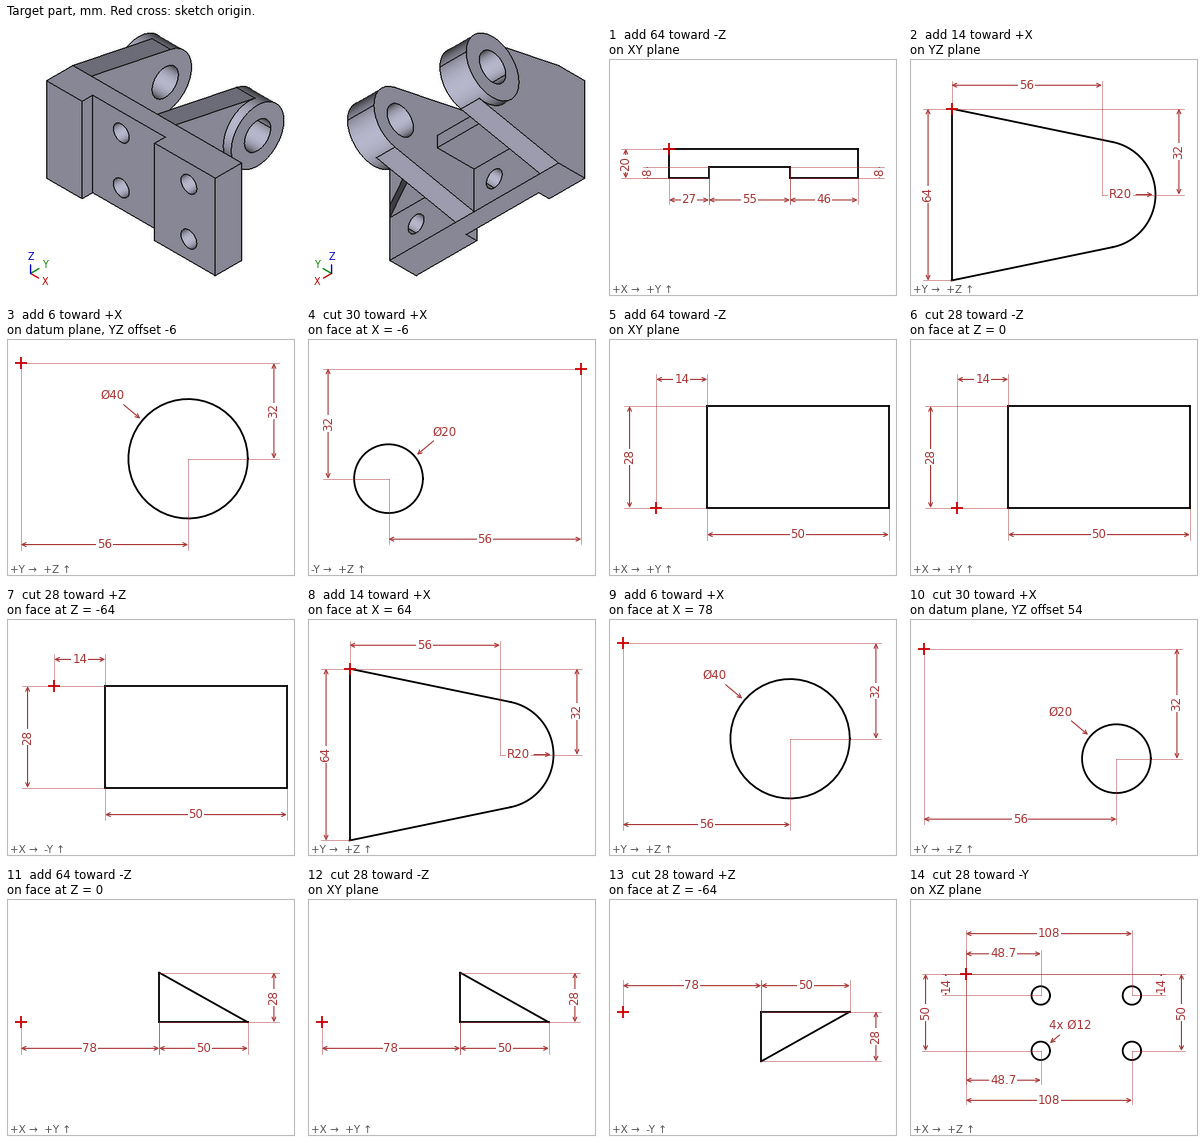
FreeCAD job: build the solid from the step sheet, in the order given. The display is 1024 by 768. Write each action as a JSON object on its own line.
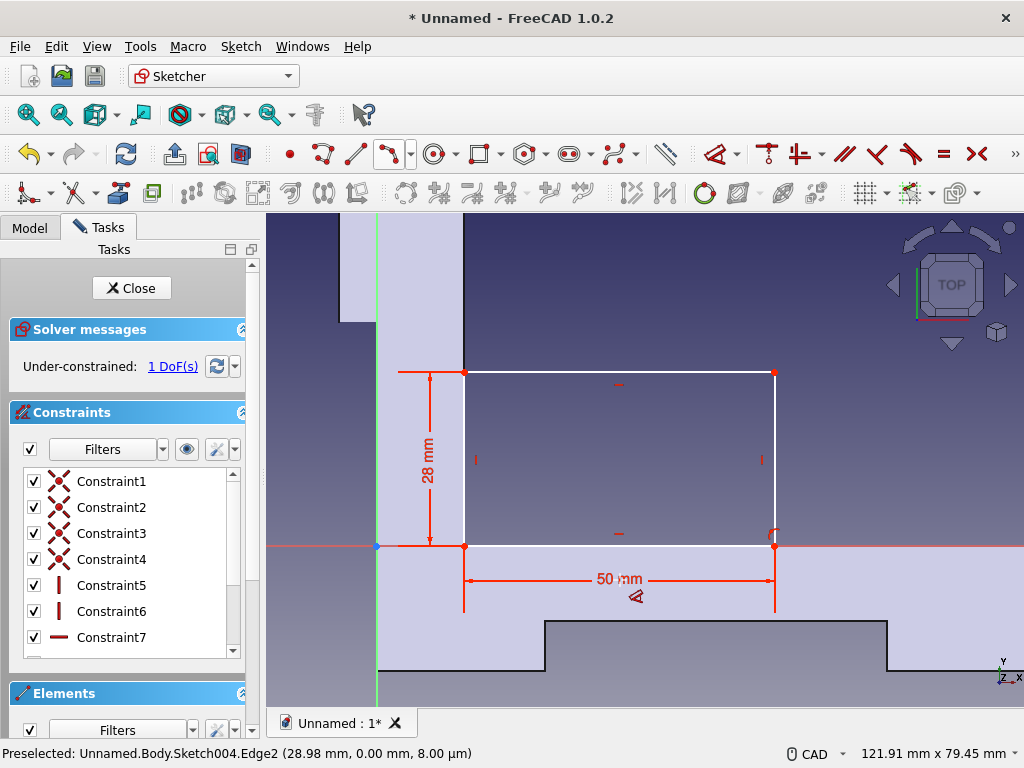
{"action": "left_click", "coordinate": [464, 372]}
{"action": "left_click", "coordinate": [420, 580]}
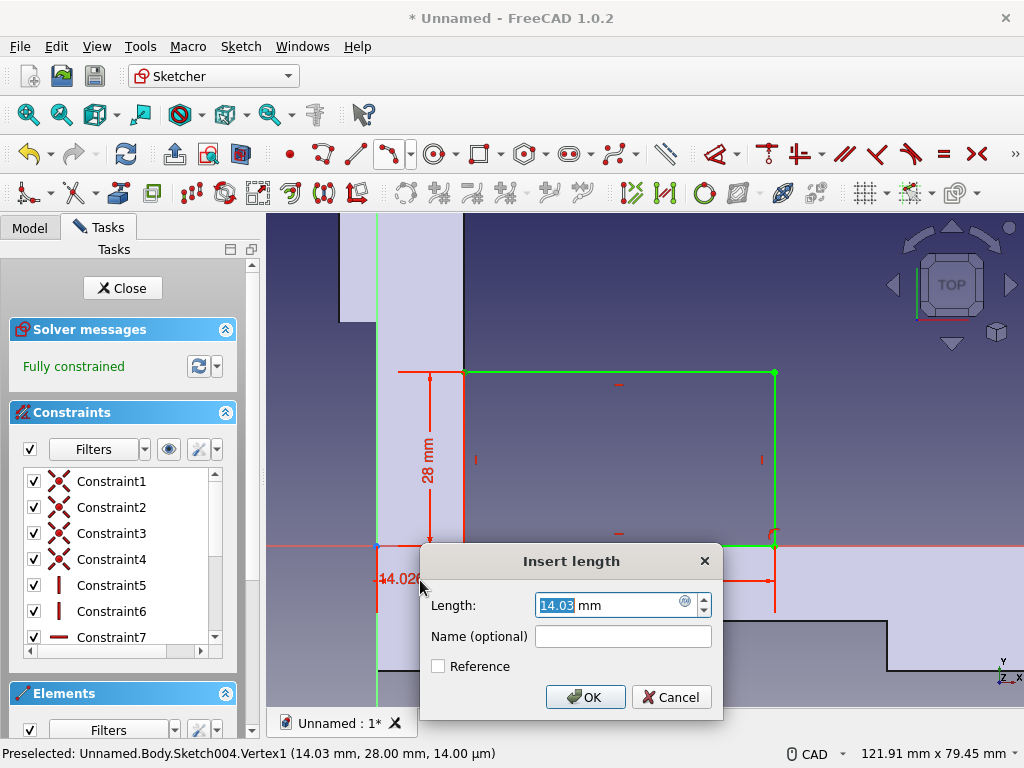
{"action": "type", "text": "14"}
{"action": "key", "text": "Return"}
{"action": "key", "text": "Escape"}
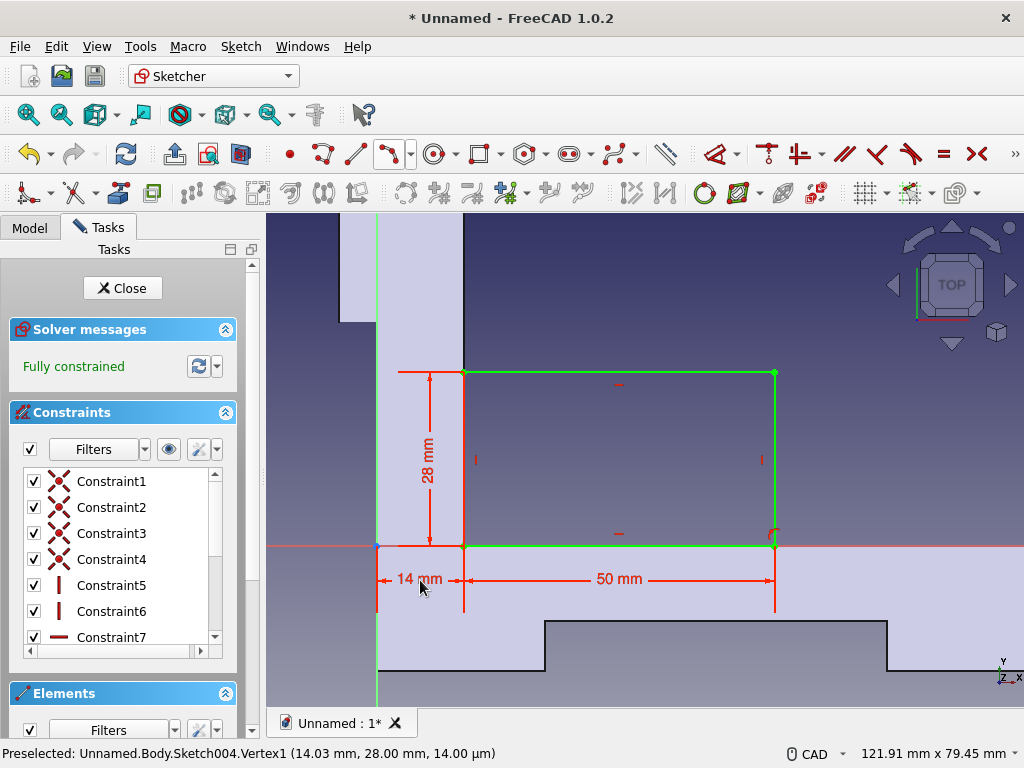
{"action": "left_click", "coordinate": [123, 288]}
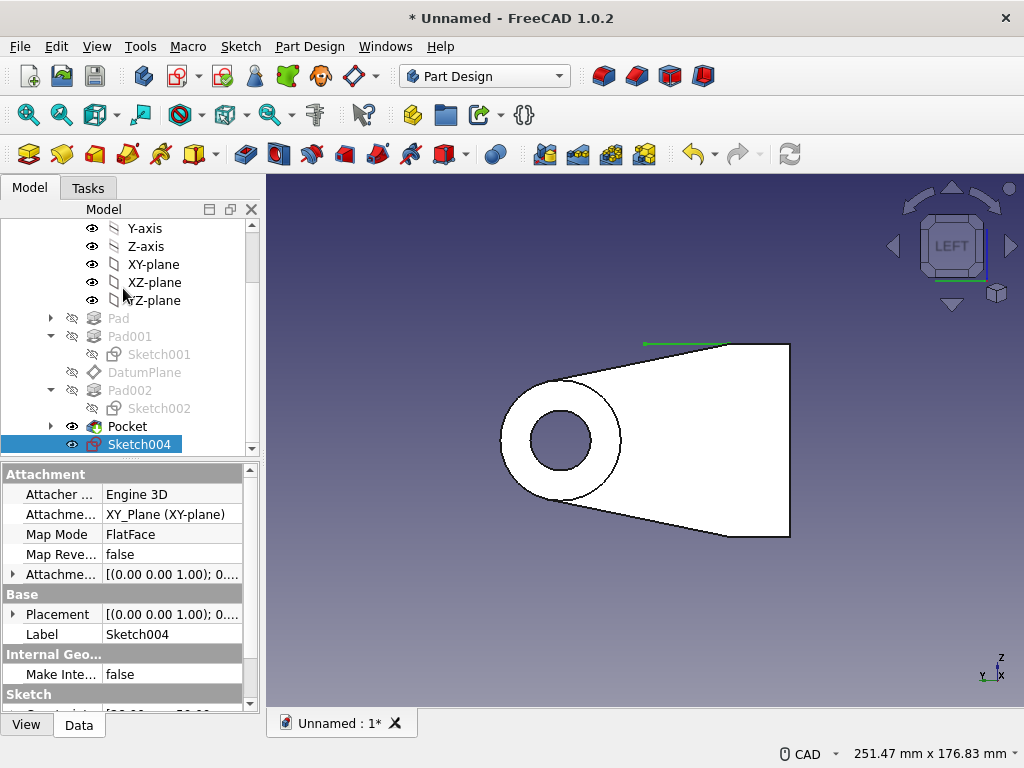
{"action": "left_click", "coordinate": [29, 154]}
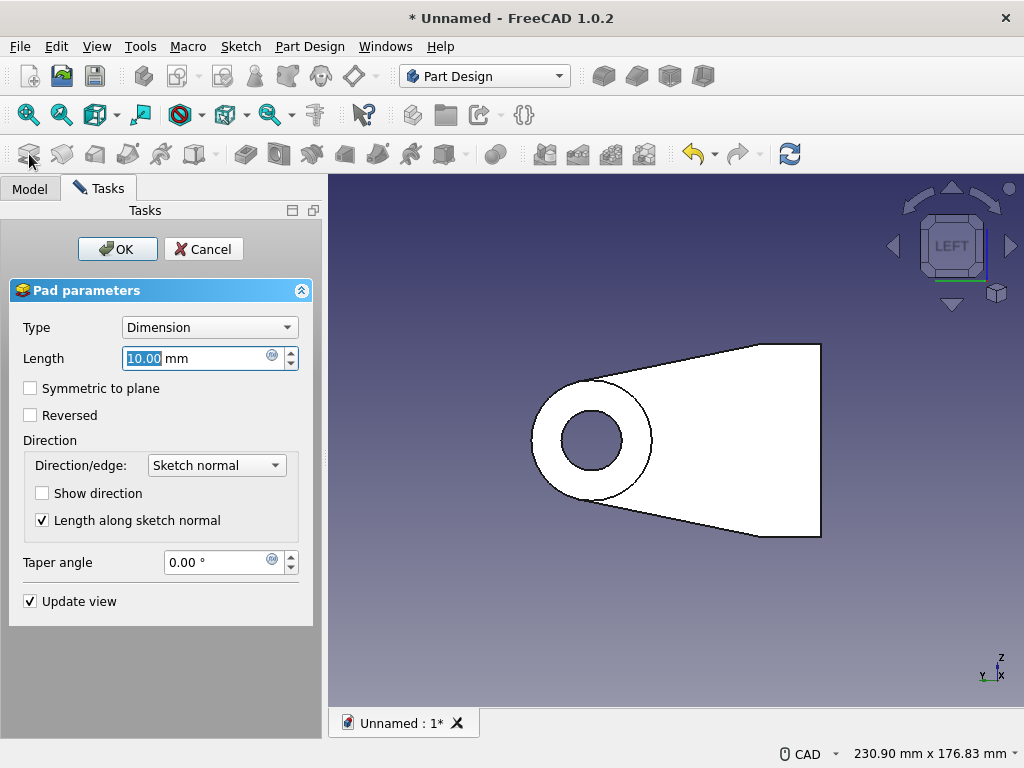
{"action": "type", "text": "64"}
{"action": "key", "text": "Tab"}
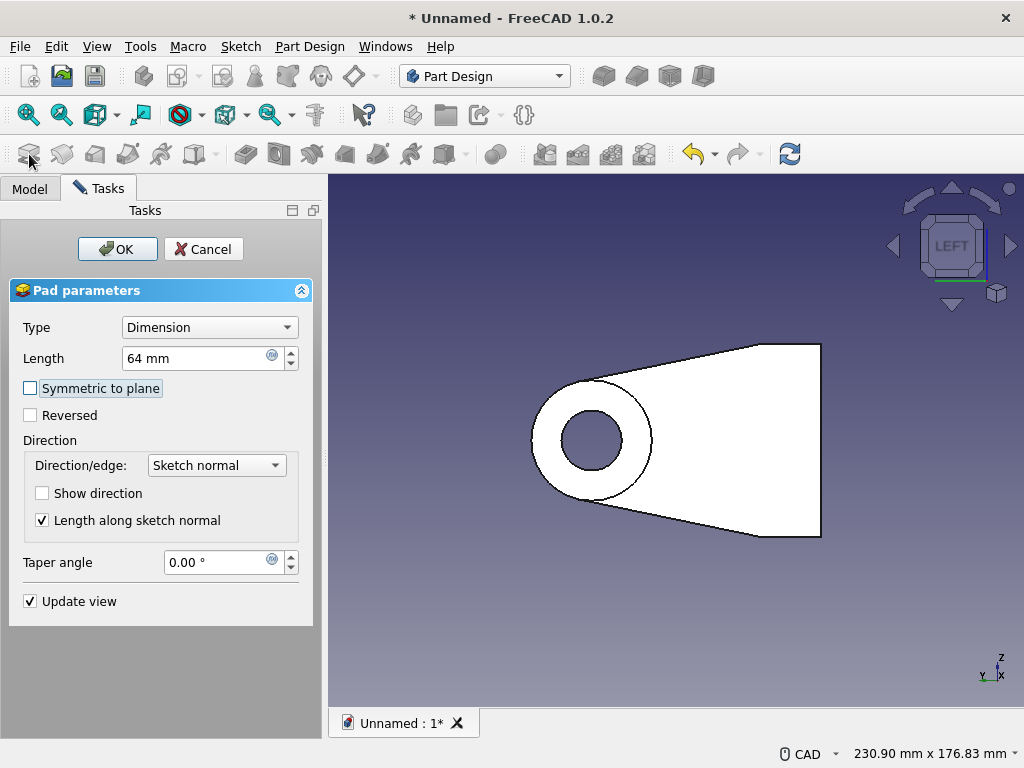
{"action": "left_click", "coordinate": [31, 415]}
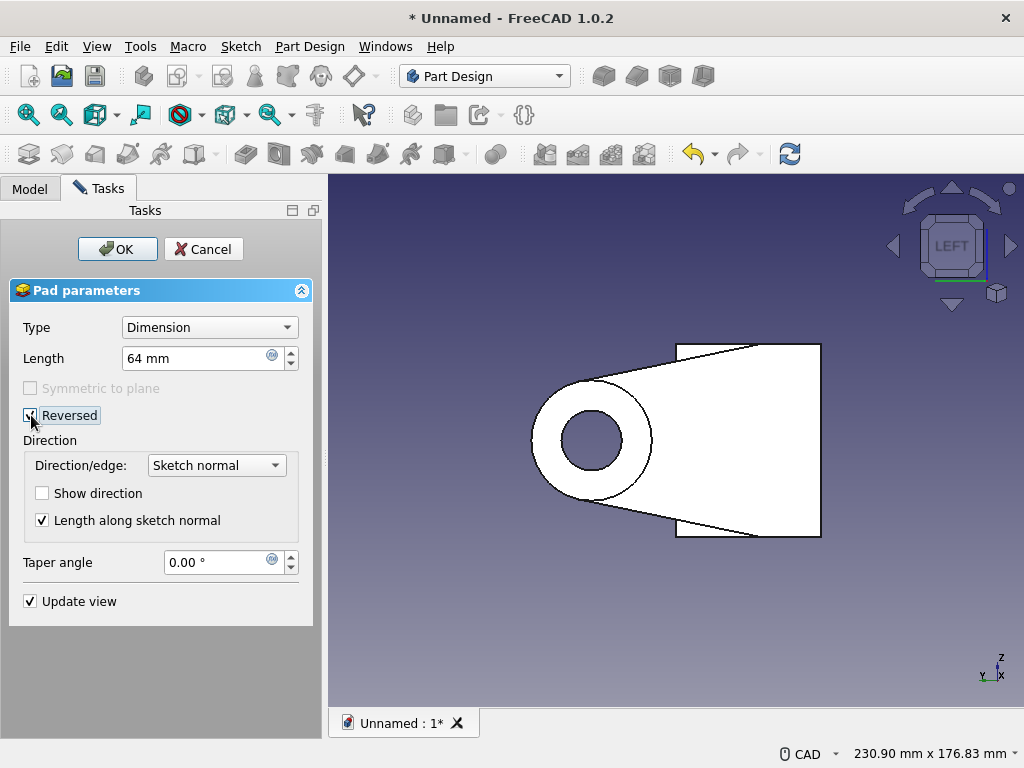
{"action": "left_click", "coordinate": [118, 249]}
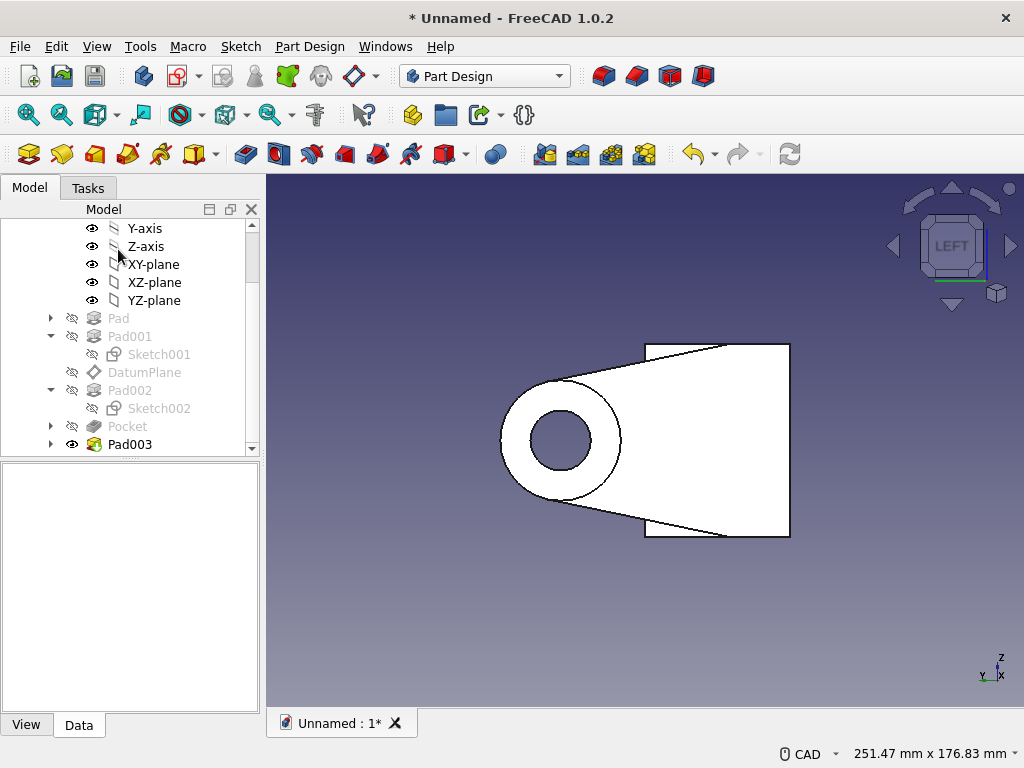
{"action": "left_click", "coordinate": [29, 116]}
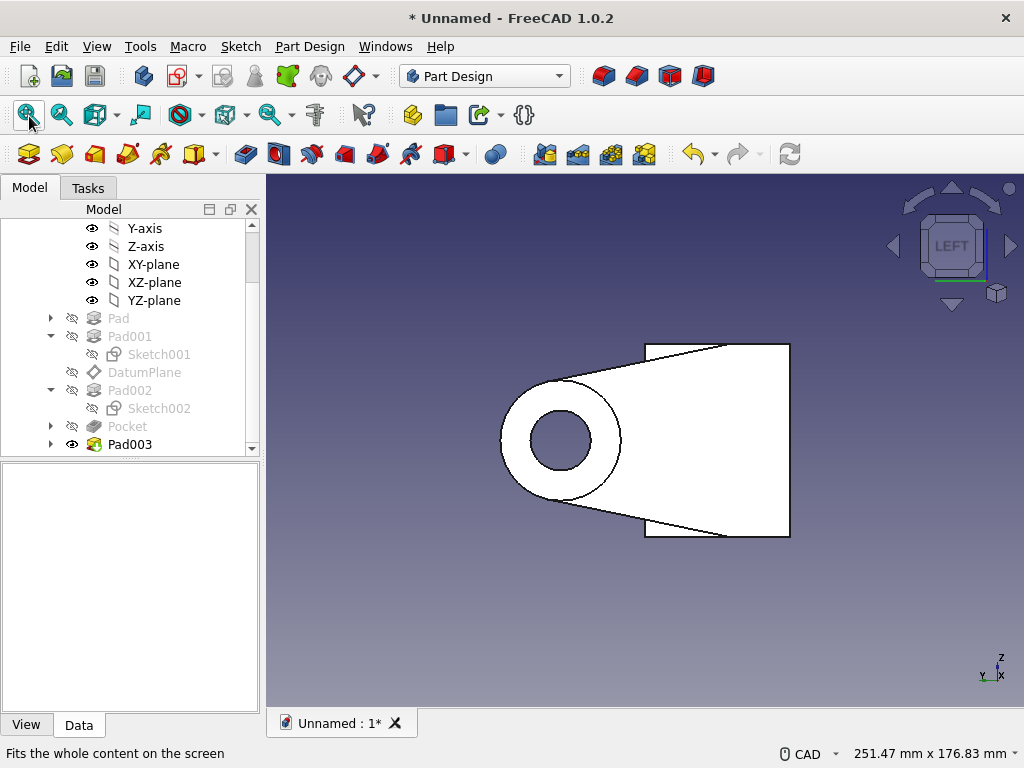
{"action": "key", "text": "0"}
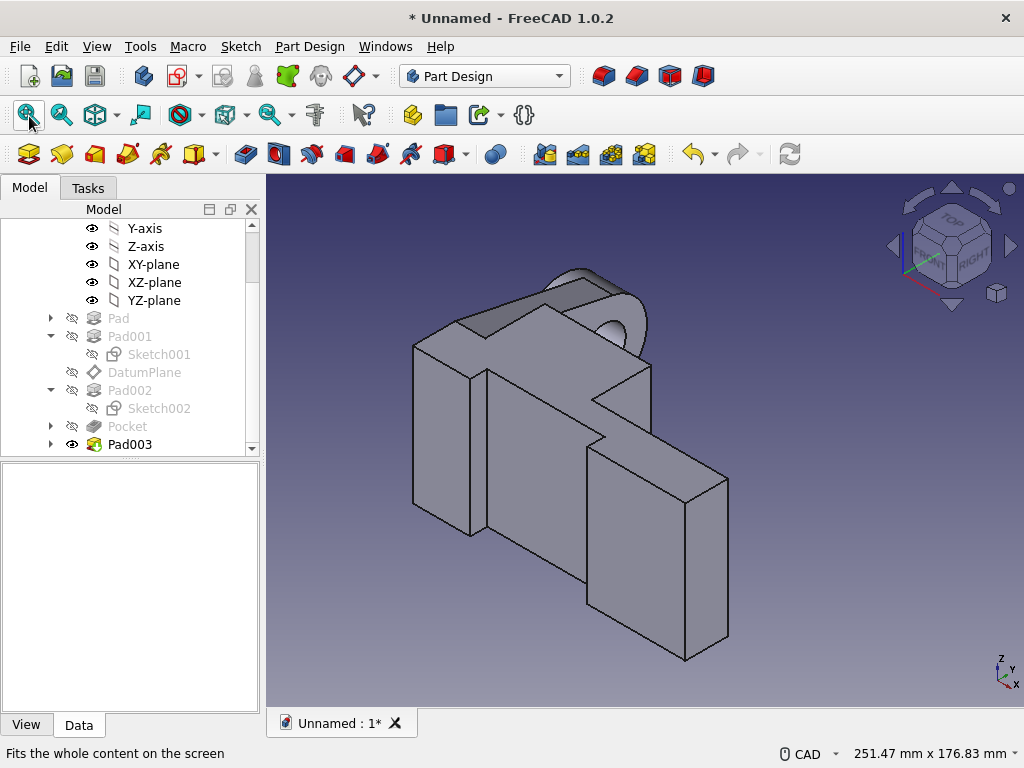
{"action": "left_click", "coordinate": [576, 363]}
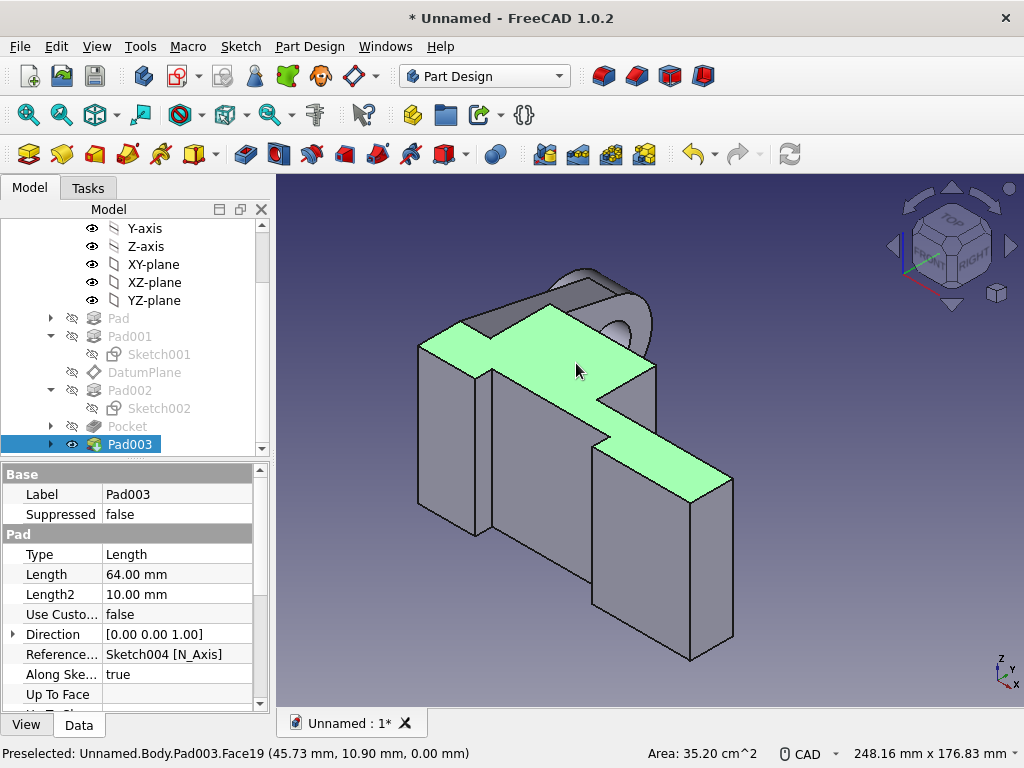
{"action": "left_click", "coordinate": [176, 76]}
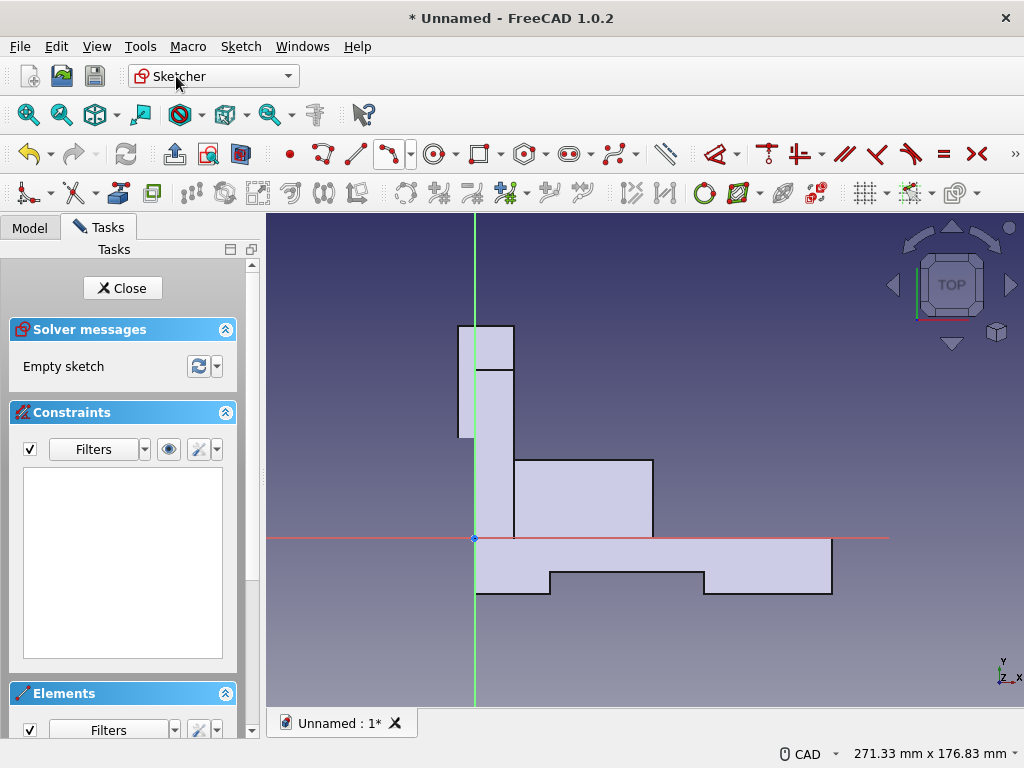
{"action": "scroll", "coordinate": [554, 531], "scroll_direction": "up", "scroll_amount": 4}